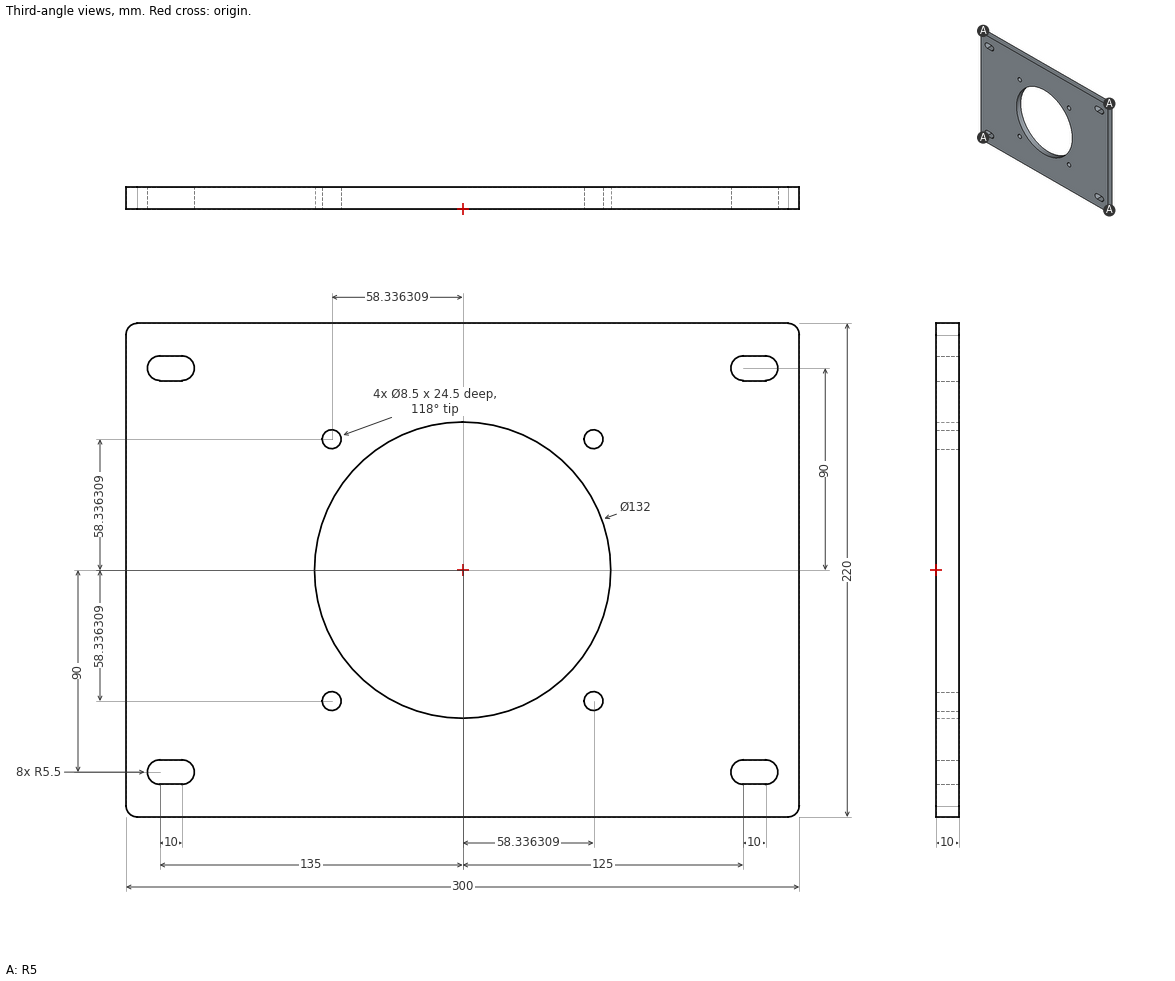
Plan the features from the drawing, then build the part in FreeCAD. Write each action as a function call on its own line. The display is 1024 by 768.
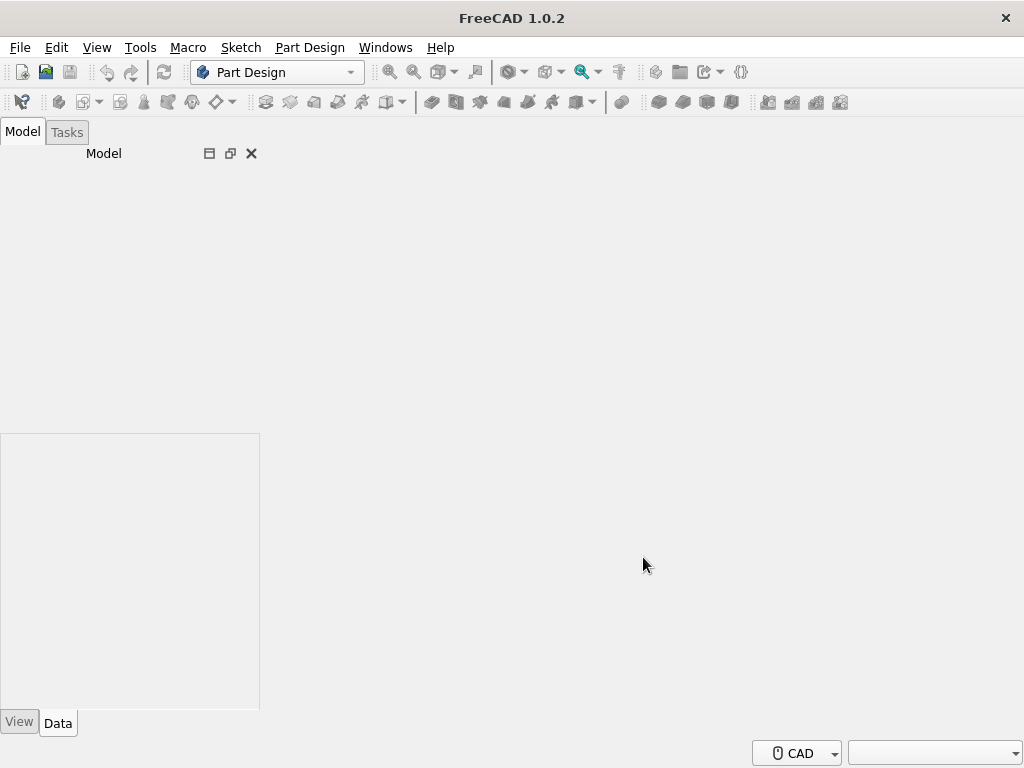
key(ctrl+n)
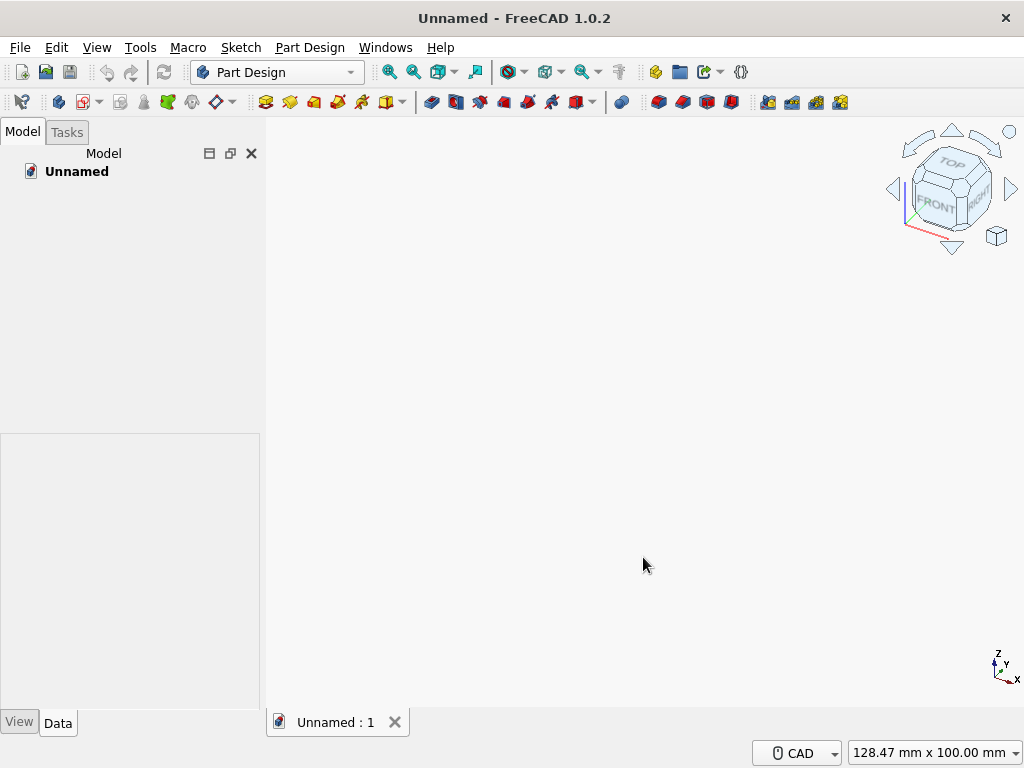
click(84, 102)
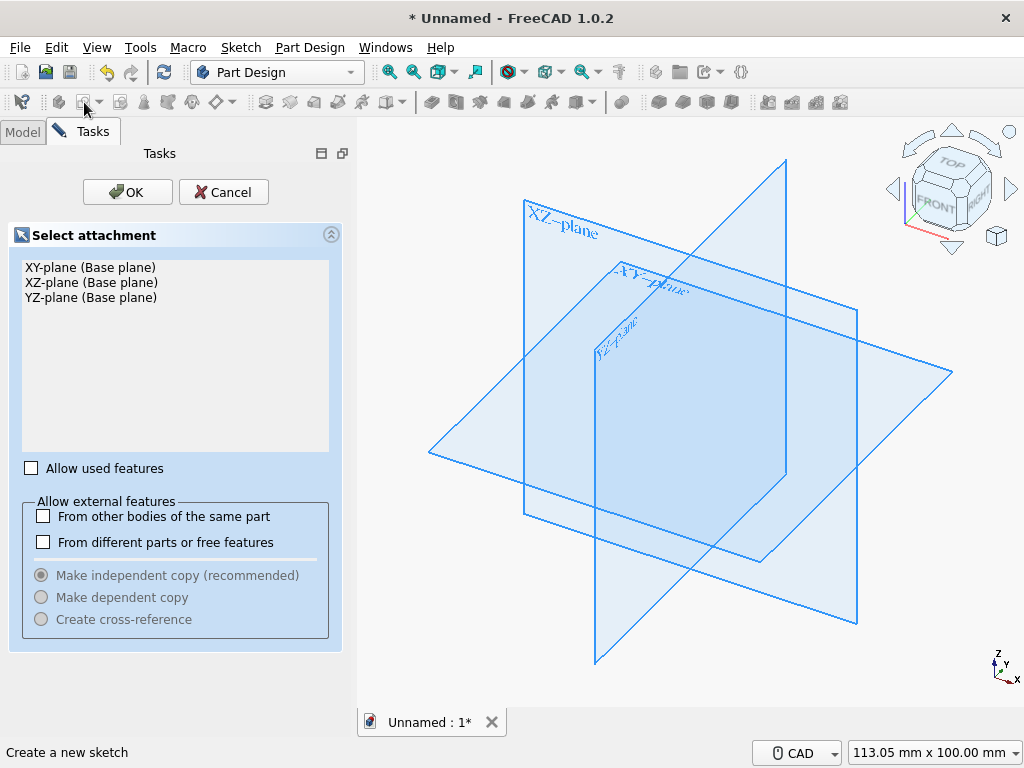
click(82, 282)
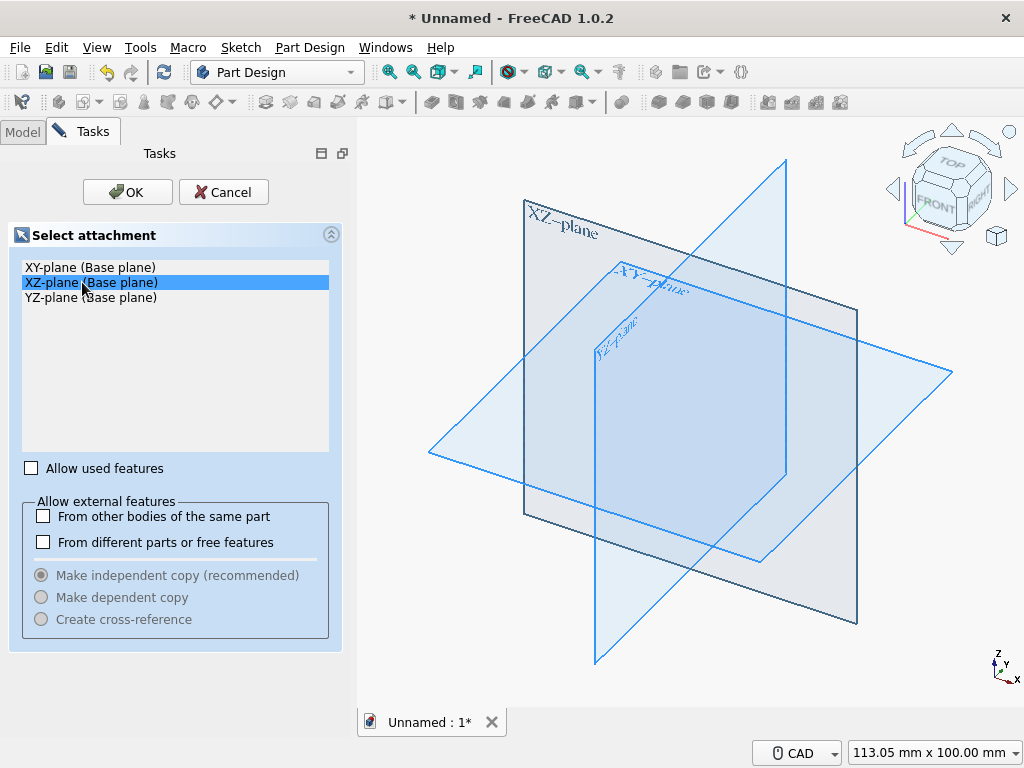
click(128, 192)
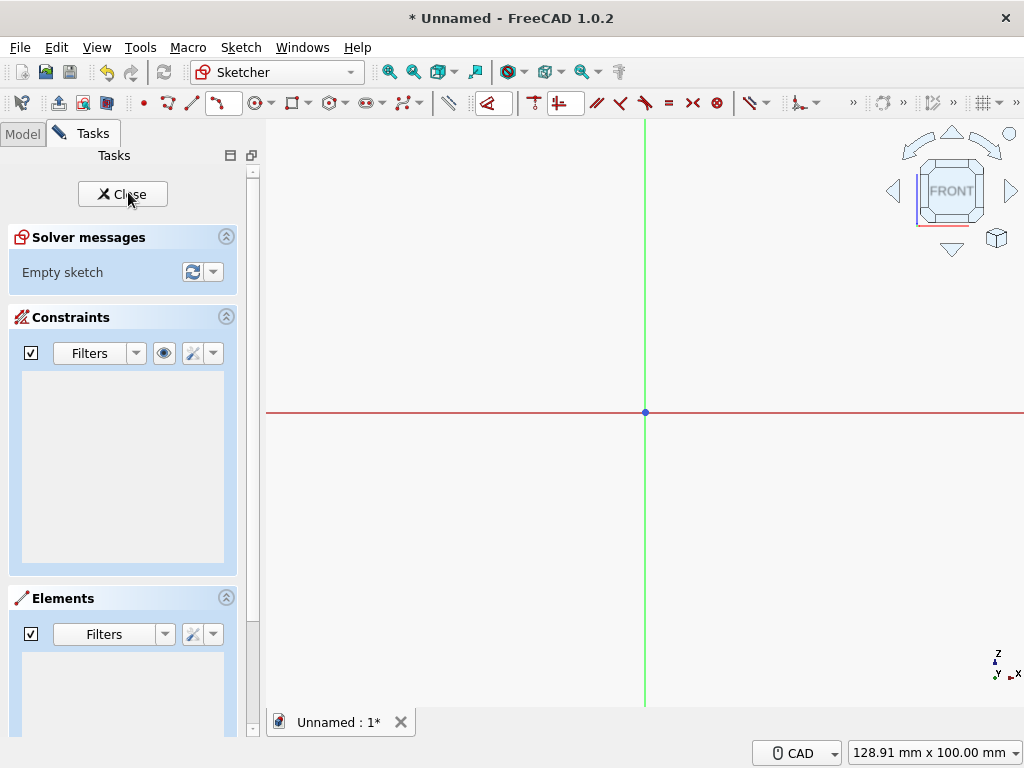
scroll(554, 413, down, 7)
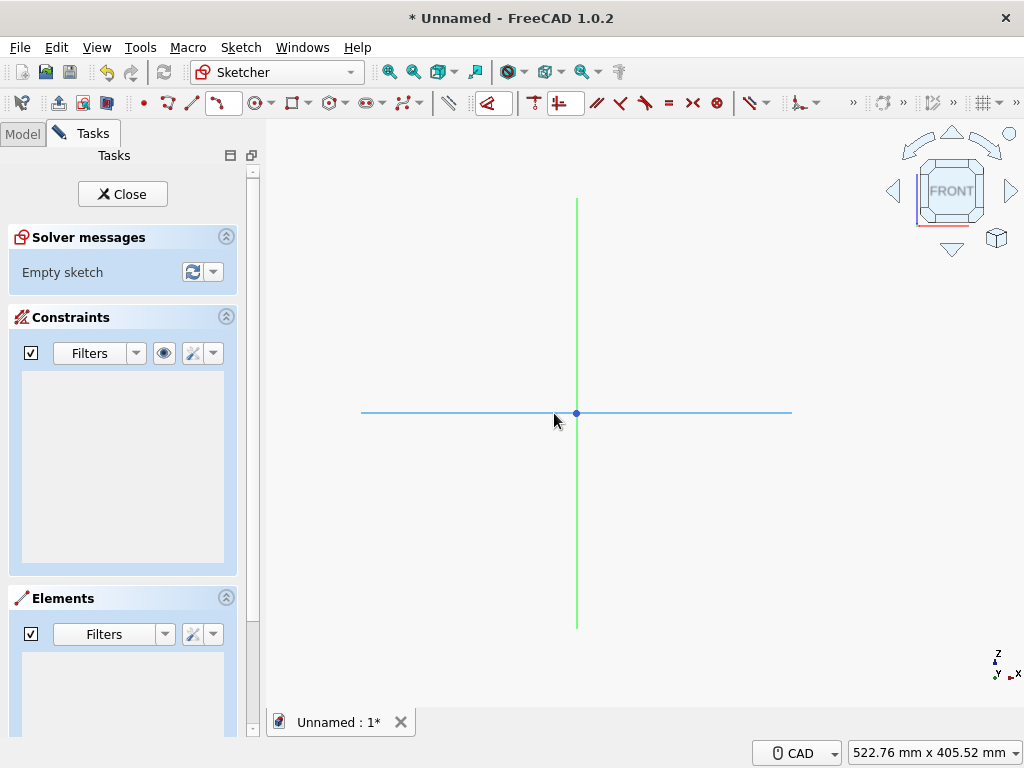
key(g)
key(v)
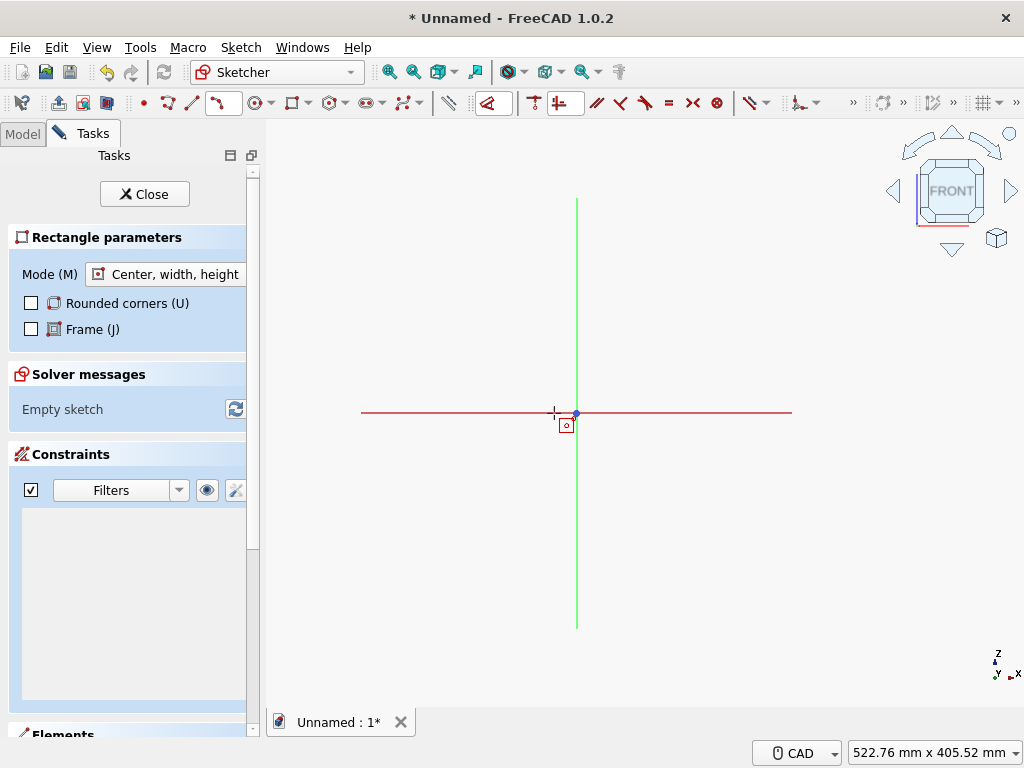
click(577, 413)
click(794, 254)
key(Escape)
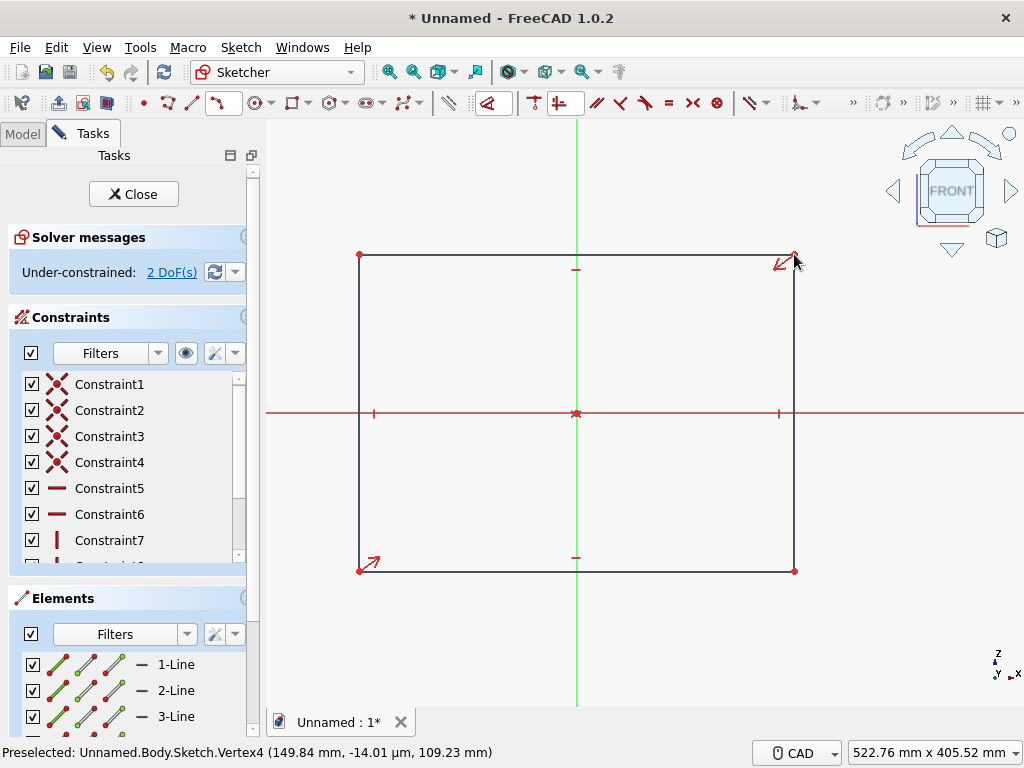
click(488, 104)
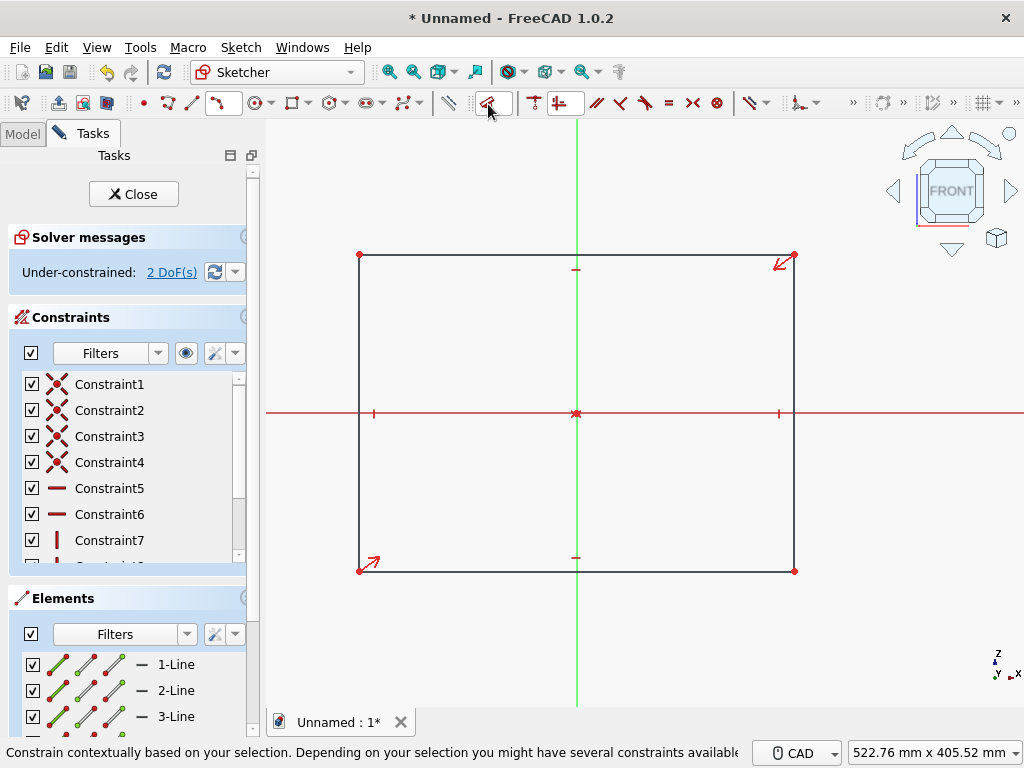
click(490, 572)
click(477, 606)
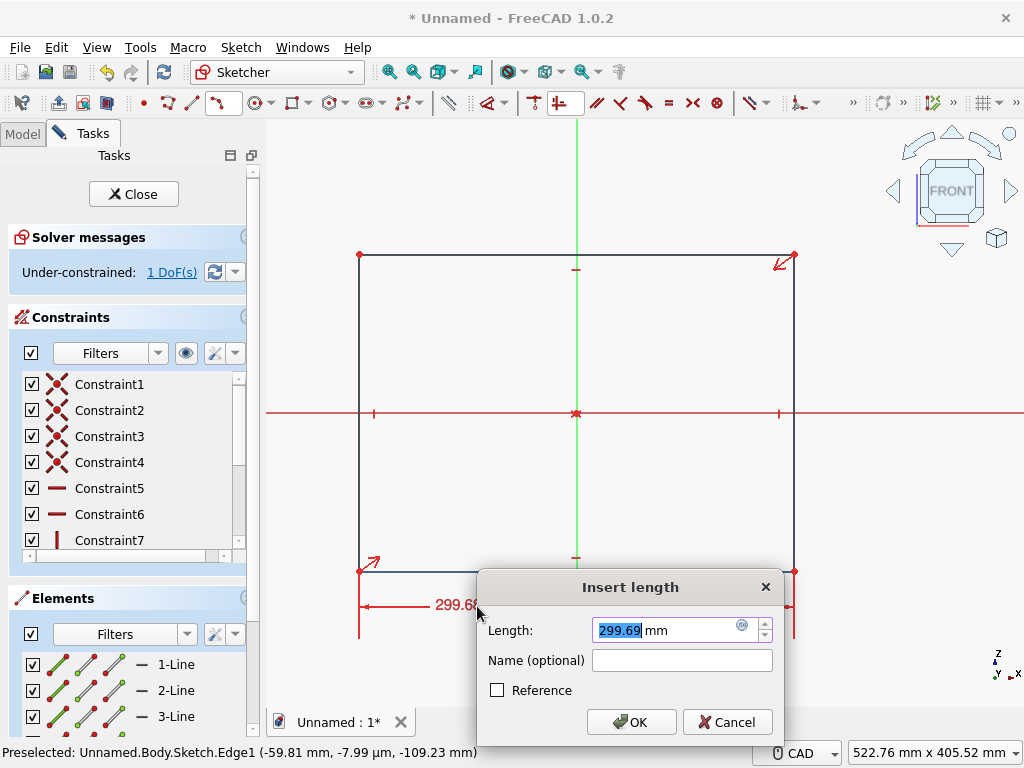
text(300)
key(Return)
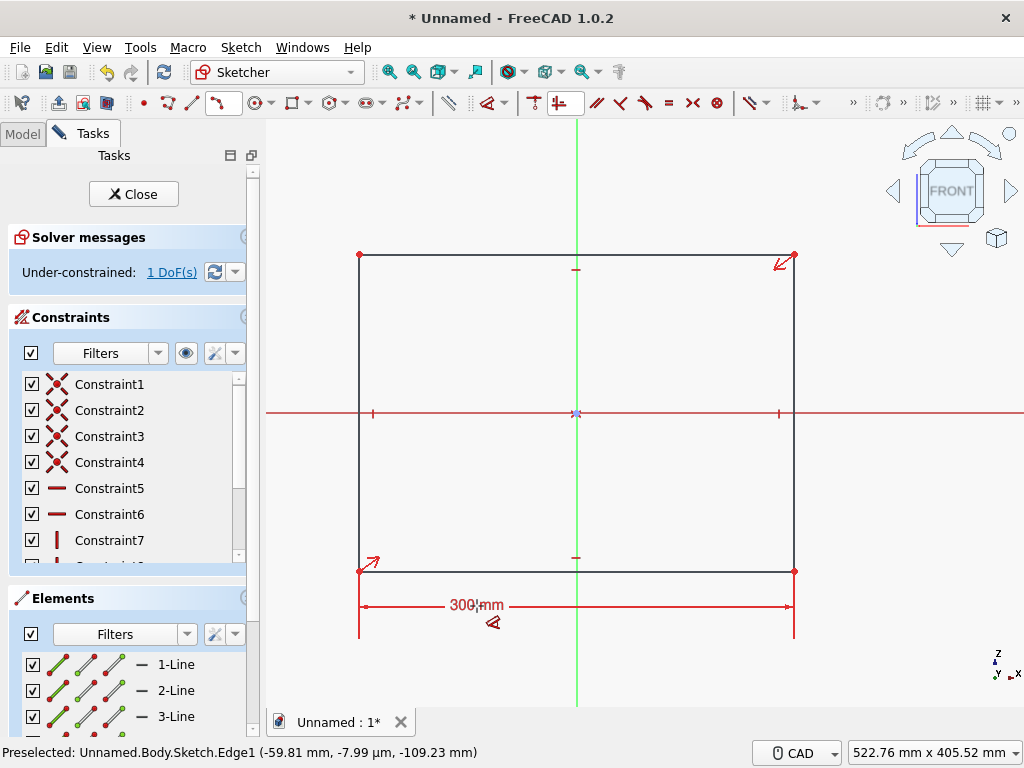
click(794, 477)
click(828, 341)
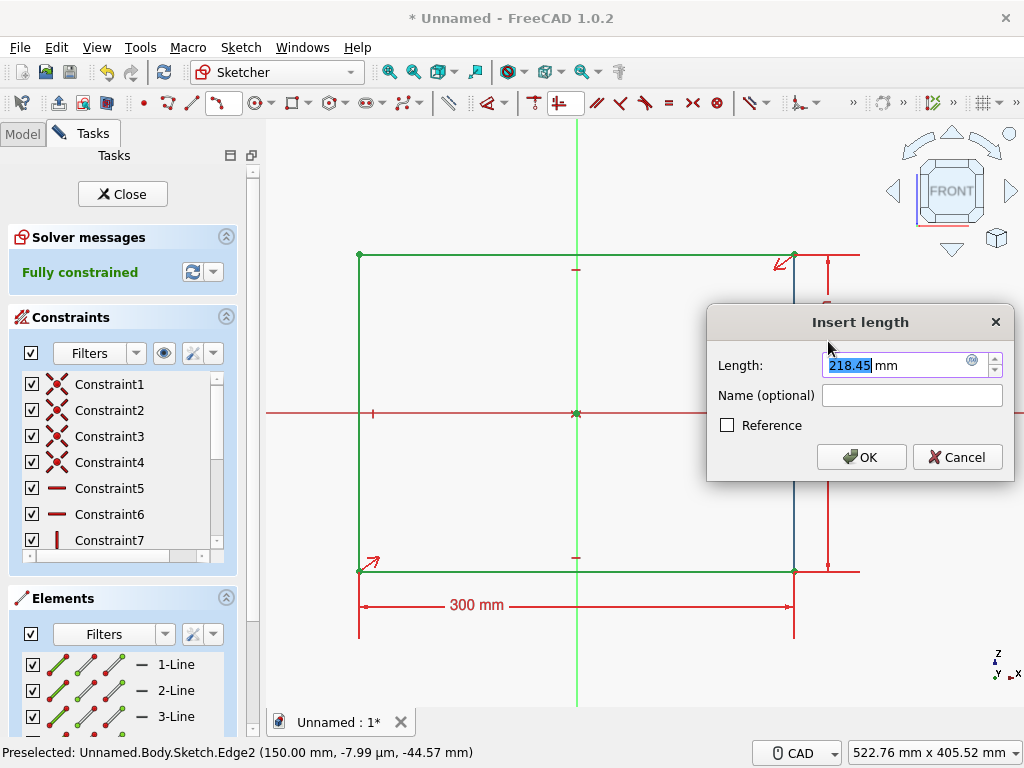
text(220)
key(Return)
key(Escape)